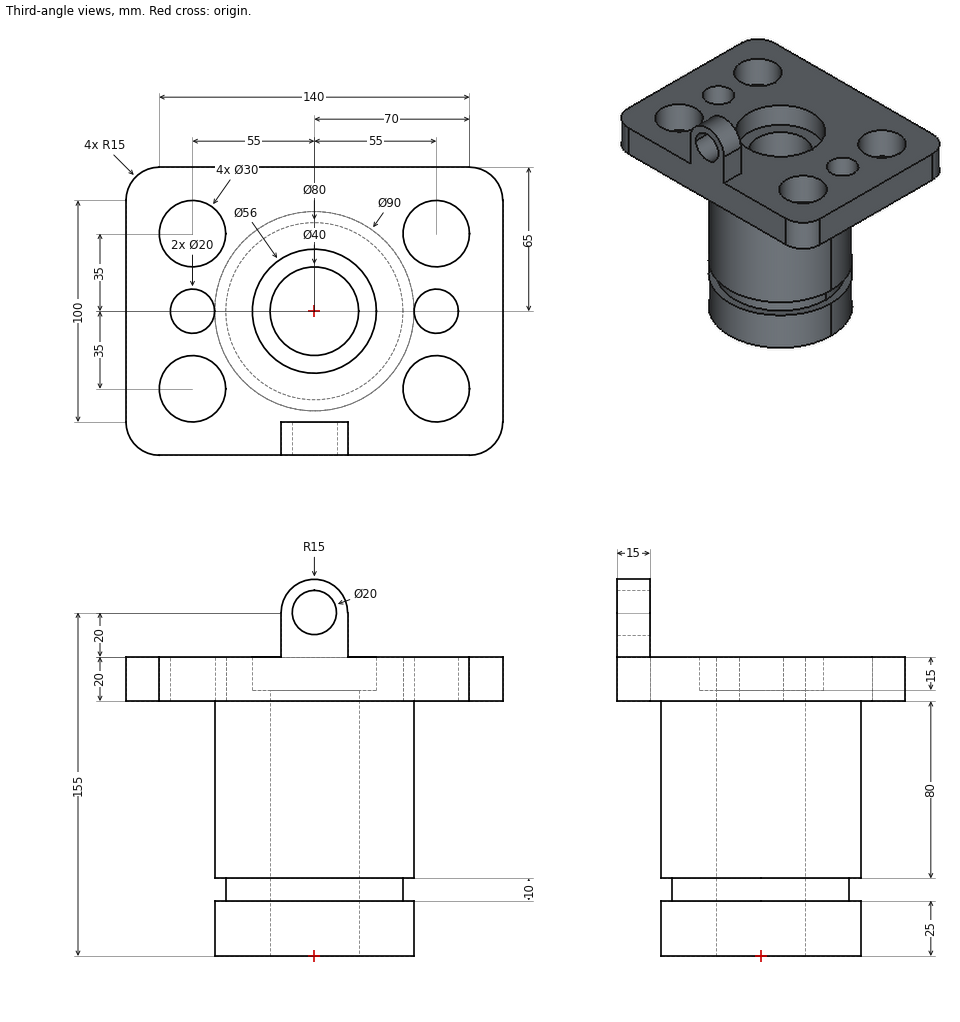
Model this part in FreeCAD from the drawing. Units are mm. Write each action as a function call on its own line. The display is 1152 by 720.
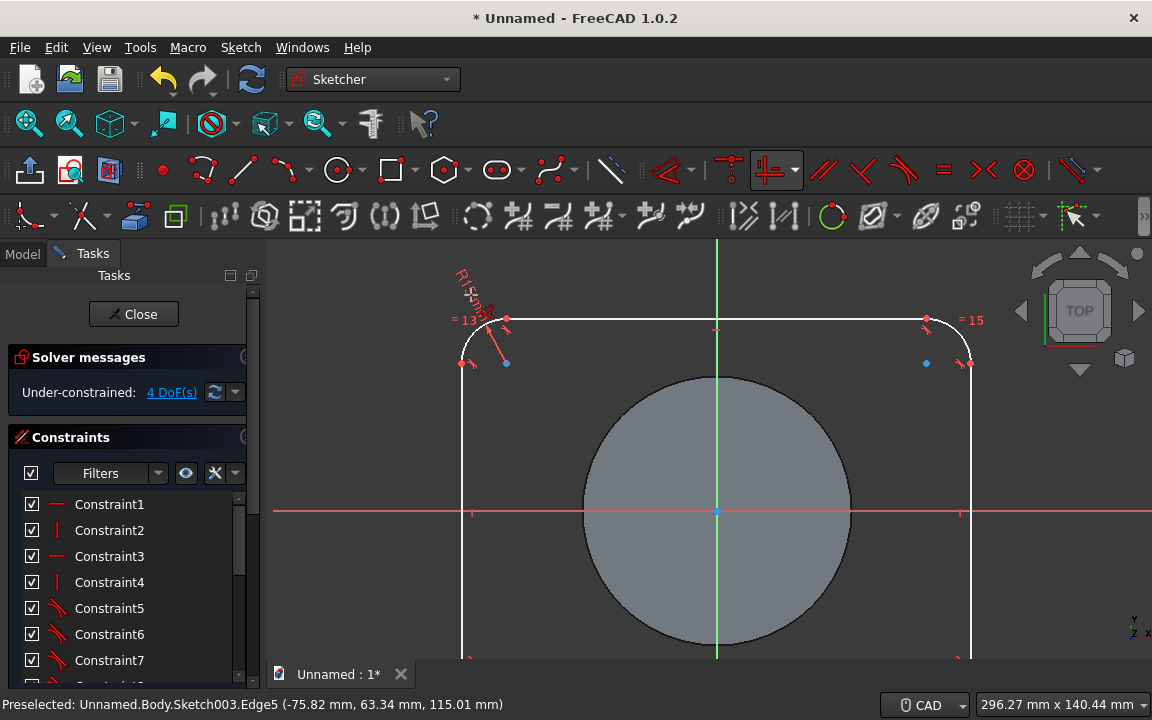
click(800, 319)
click(620, 285)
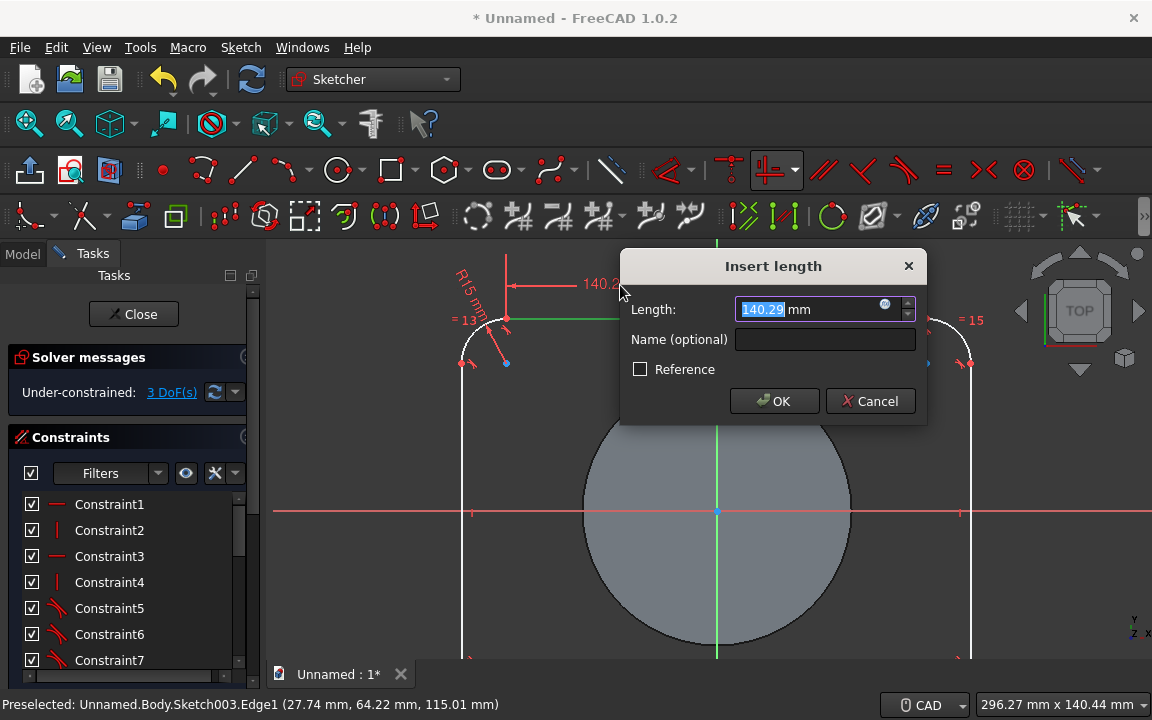
text(140)
key(Return)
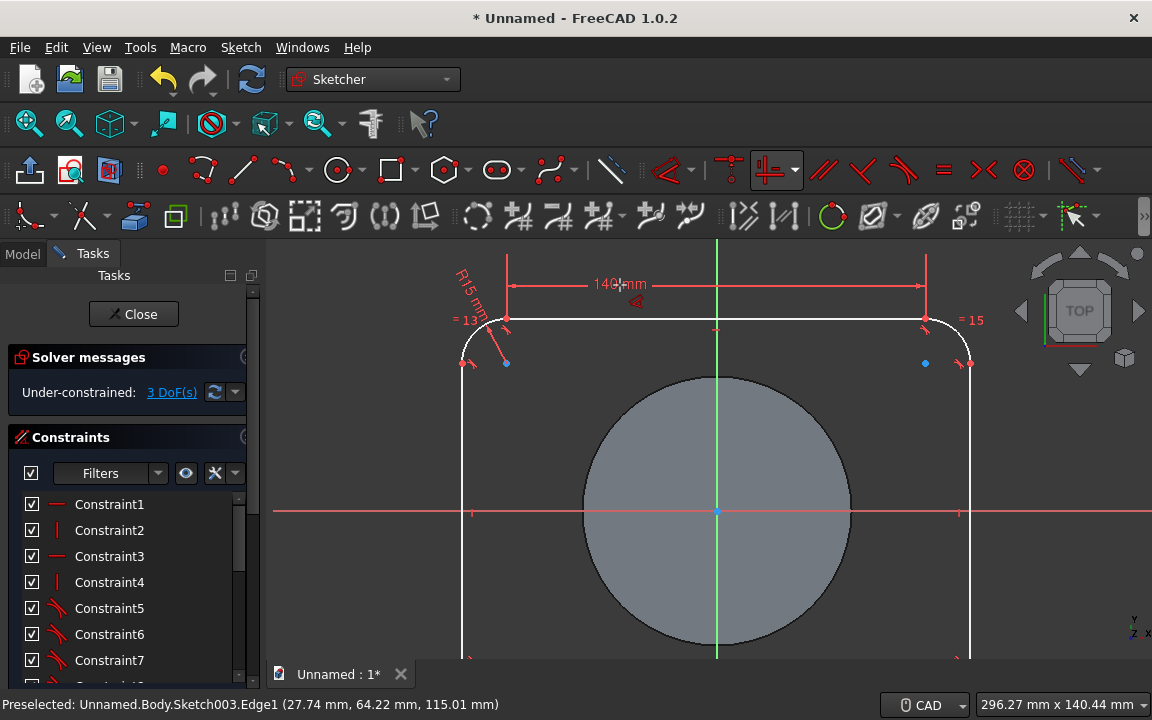
click(462, 453)
click(428, 497)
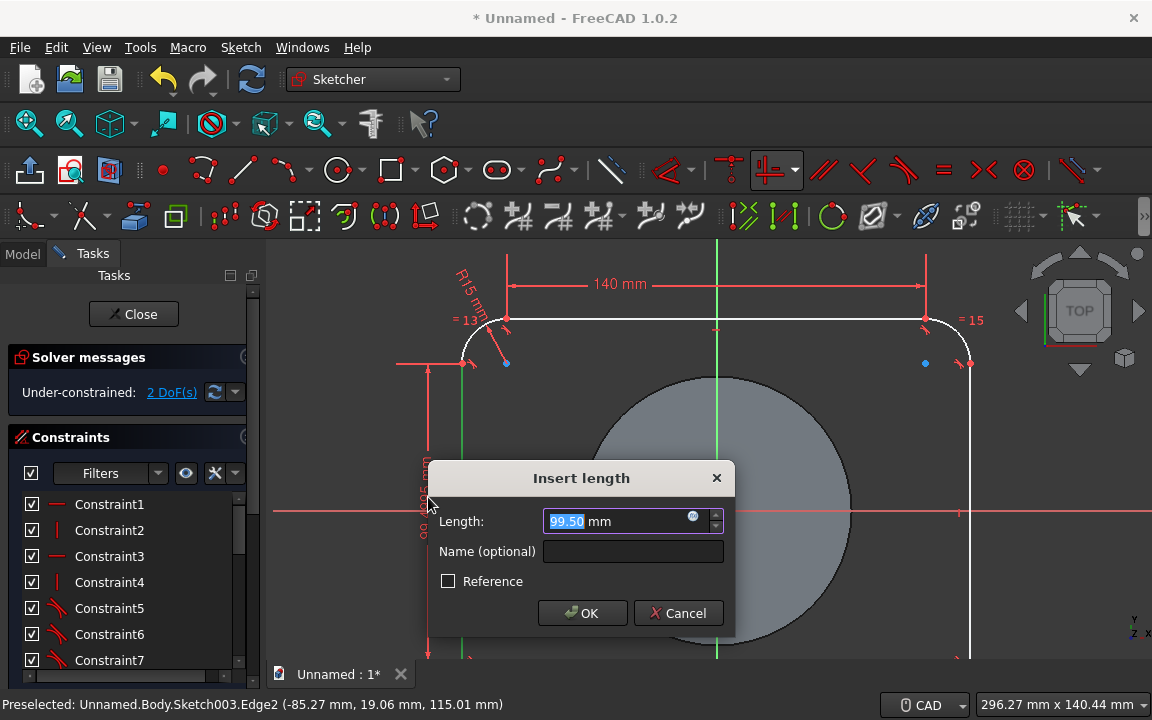
text(100)
key(Return)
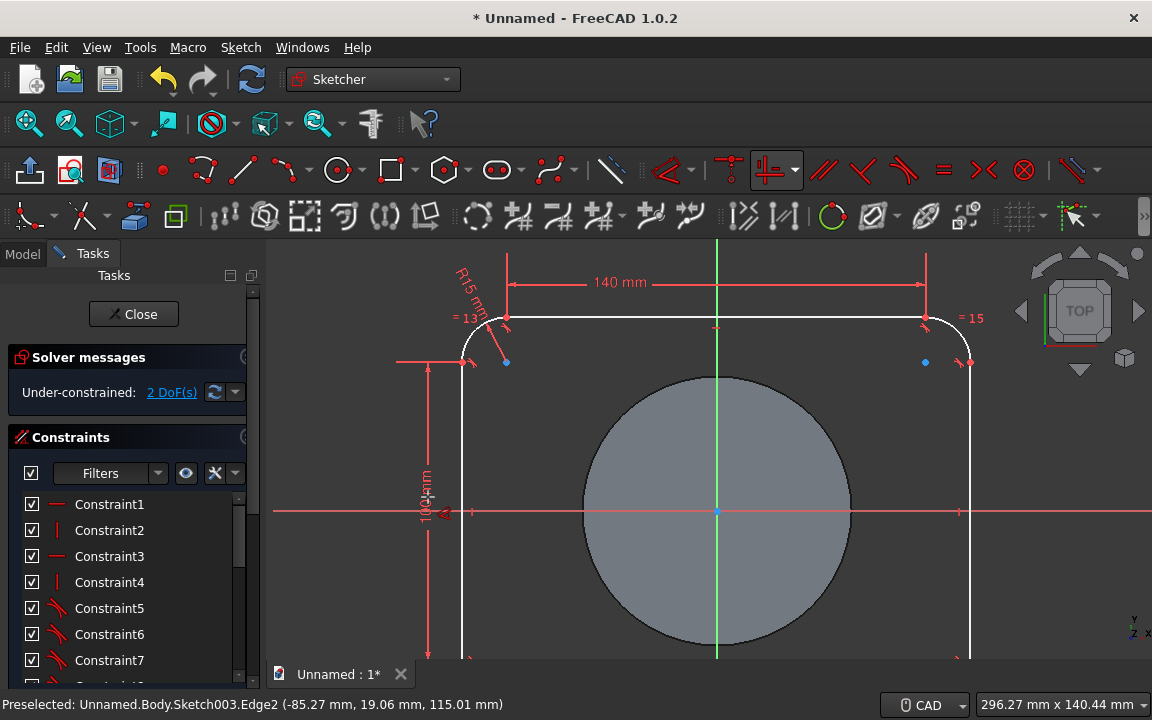
click(926, 317)
click(821, 283)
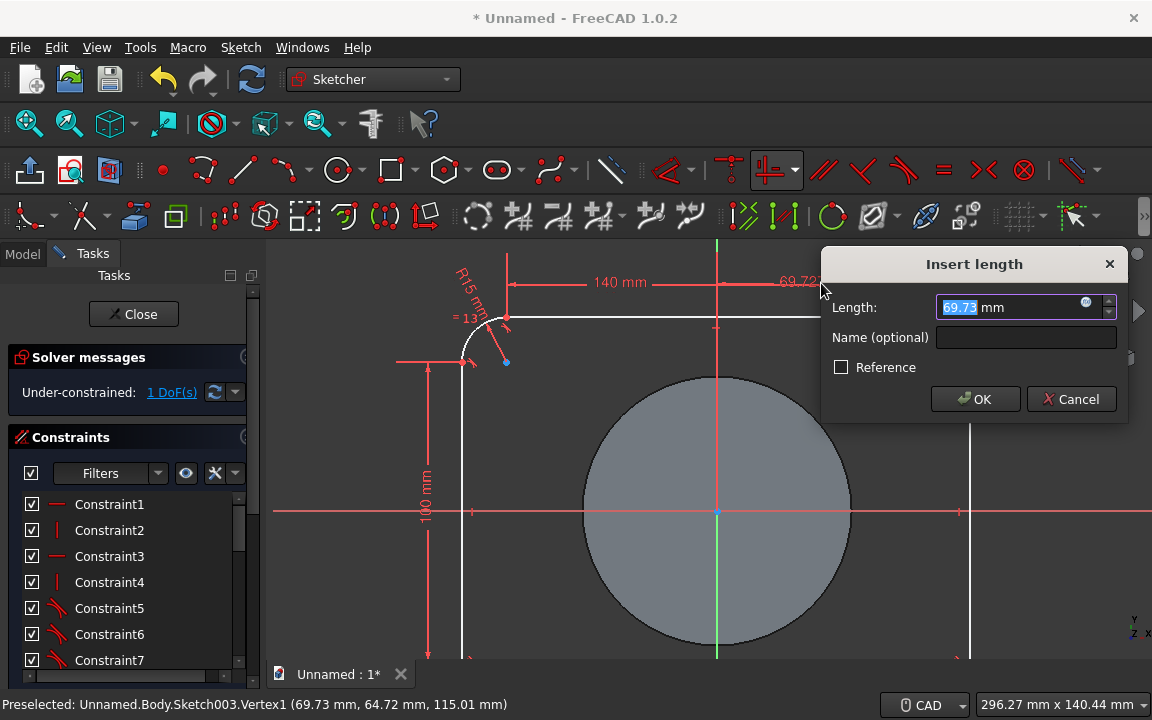
text(70)
key(Return)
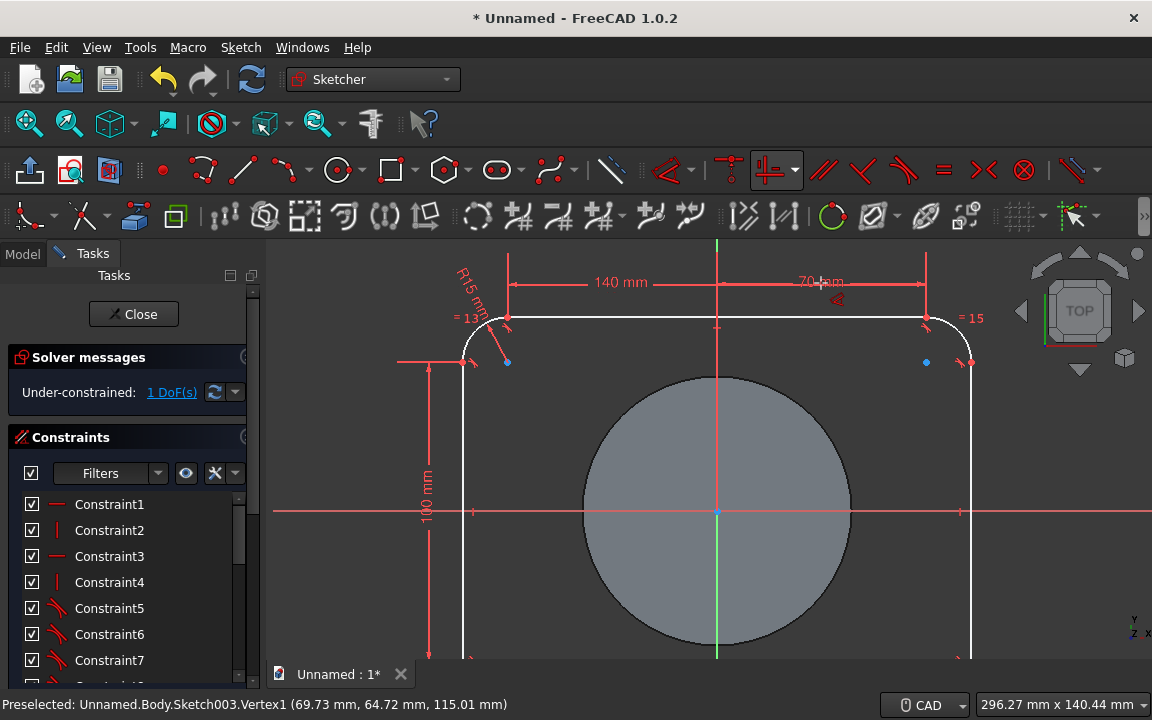
click(926, 317)
click(683, 414)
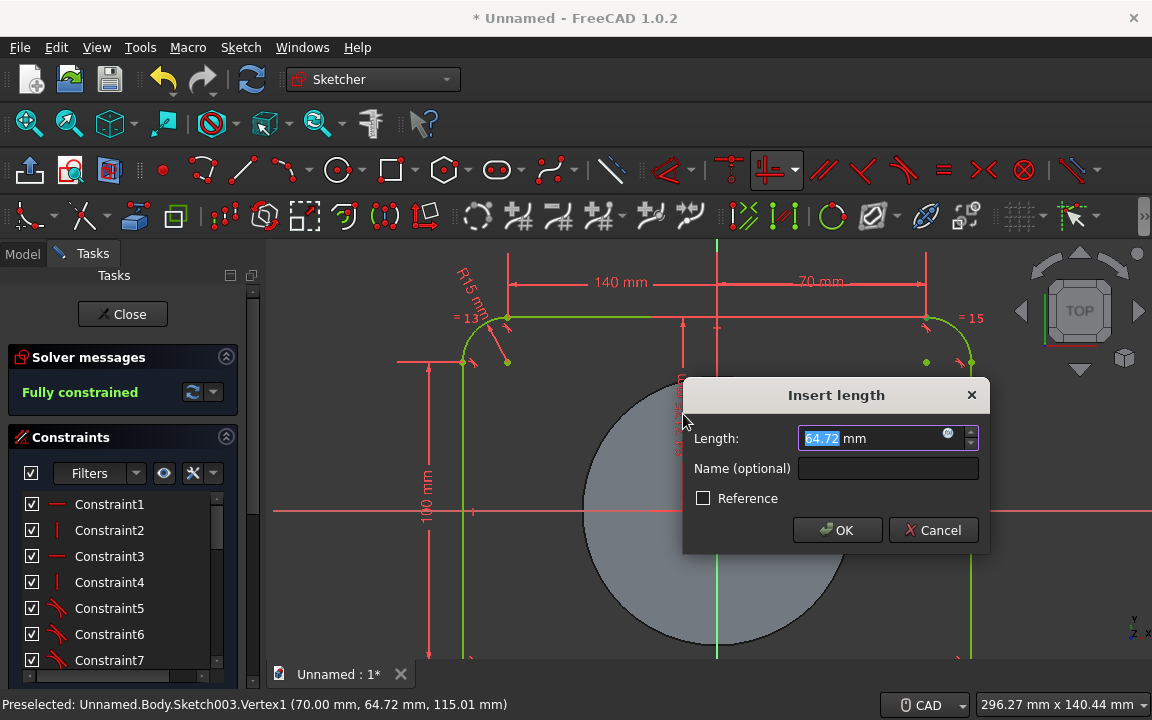
text(65)
key(Return)
key(Escape)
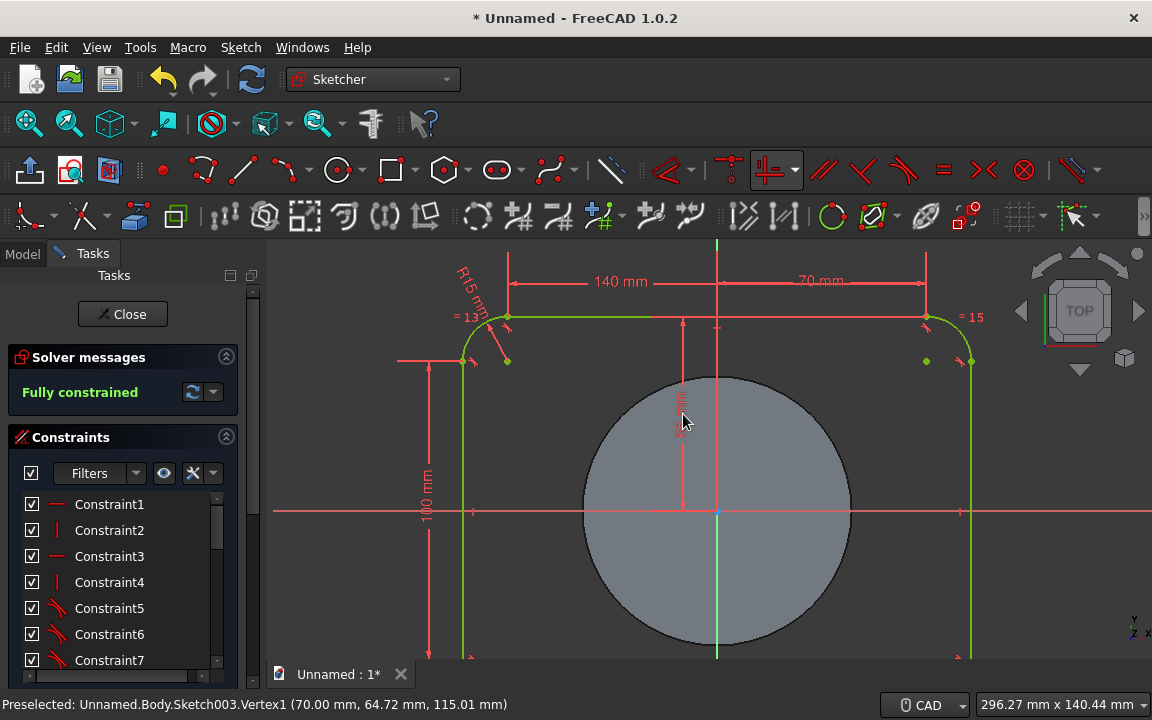
click(123, 314)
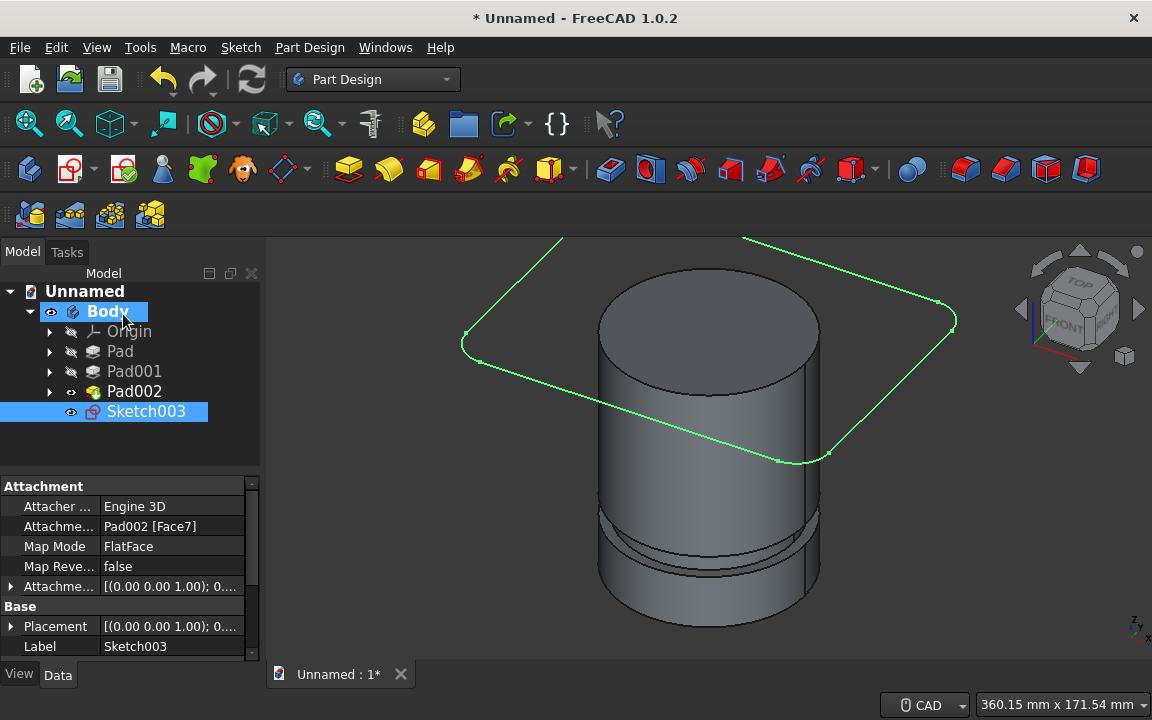
click(350, 170)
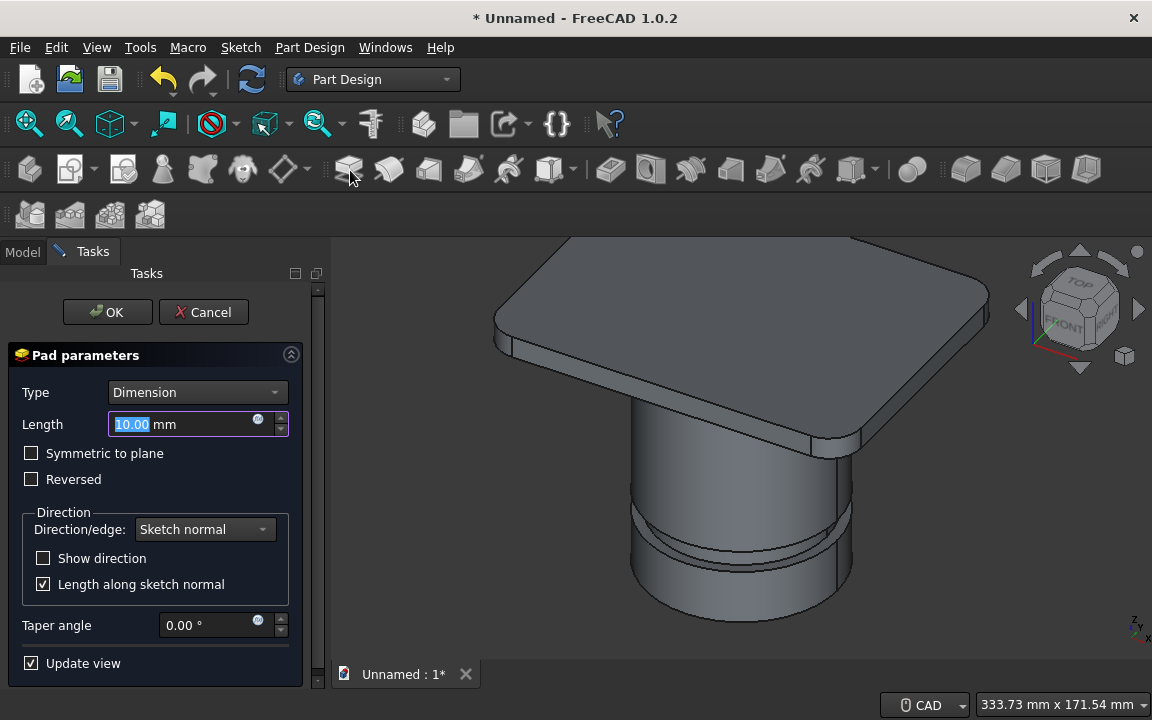
text(20)
key(Tab)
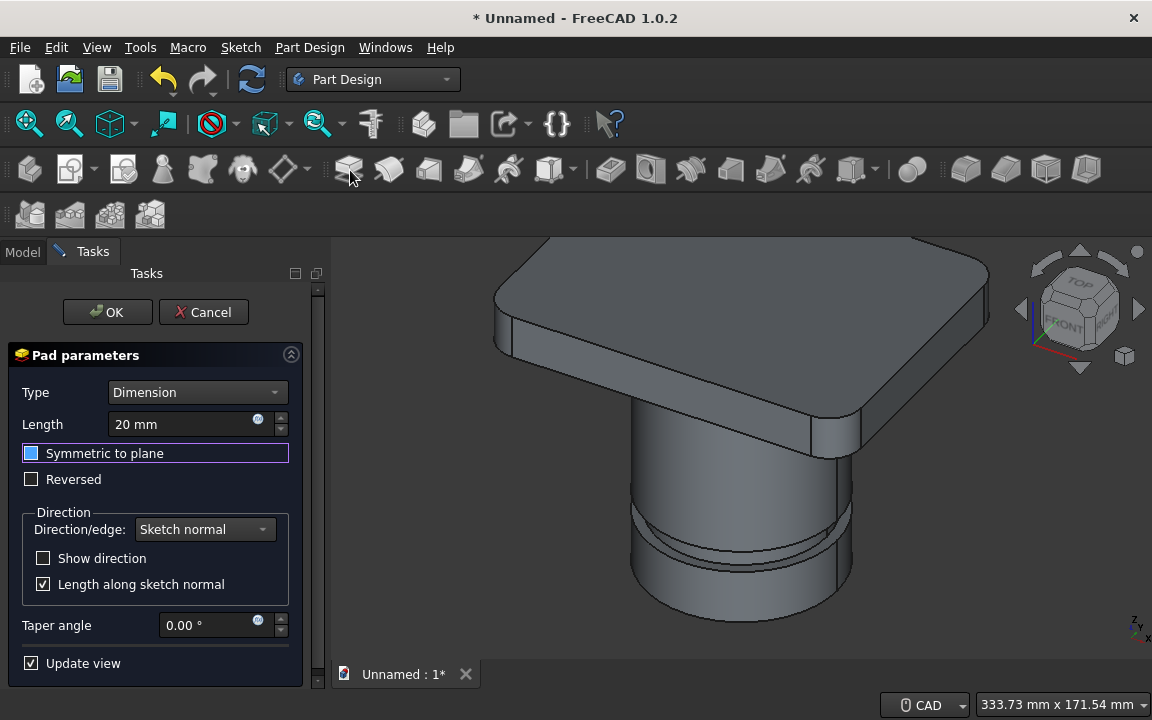
click(108, 312)